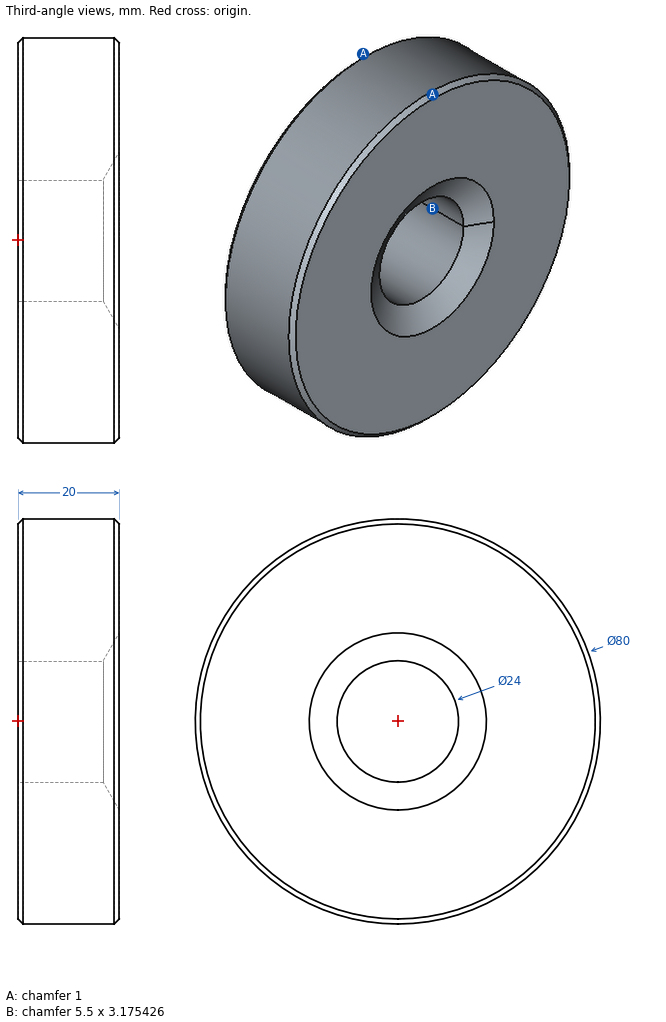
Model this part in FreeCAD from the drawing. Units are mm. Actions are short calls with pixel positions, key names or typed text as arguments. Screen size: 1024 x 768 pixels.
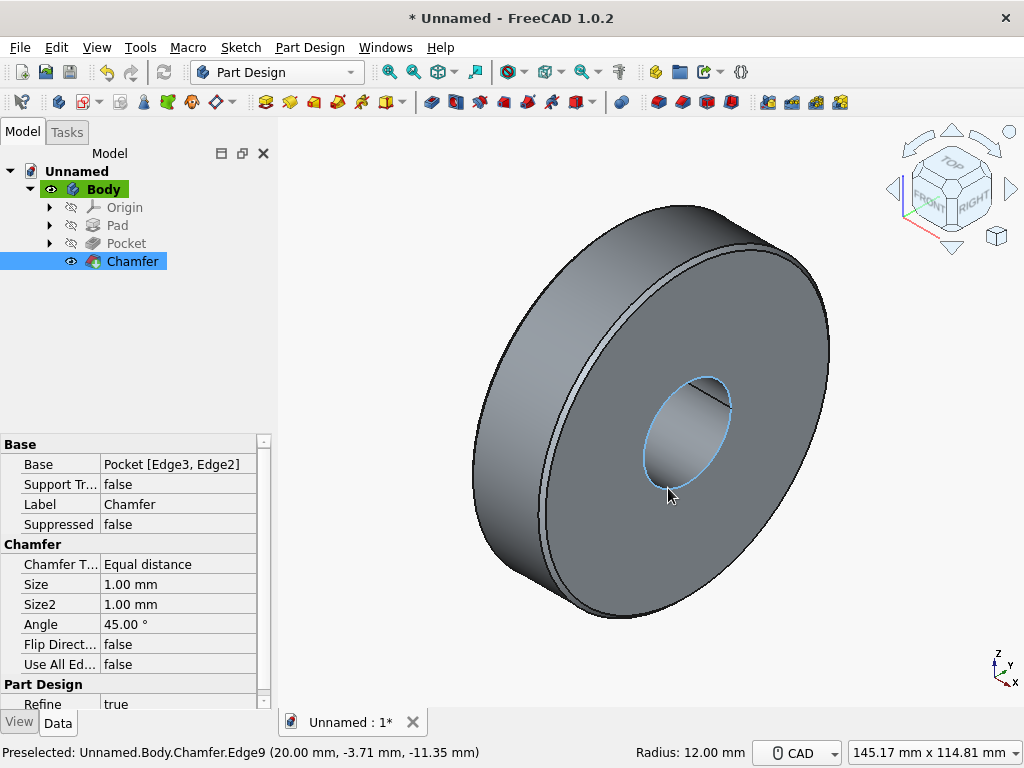
click(684, 102)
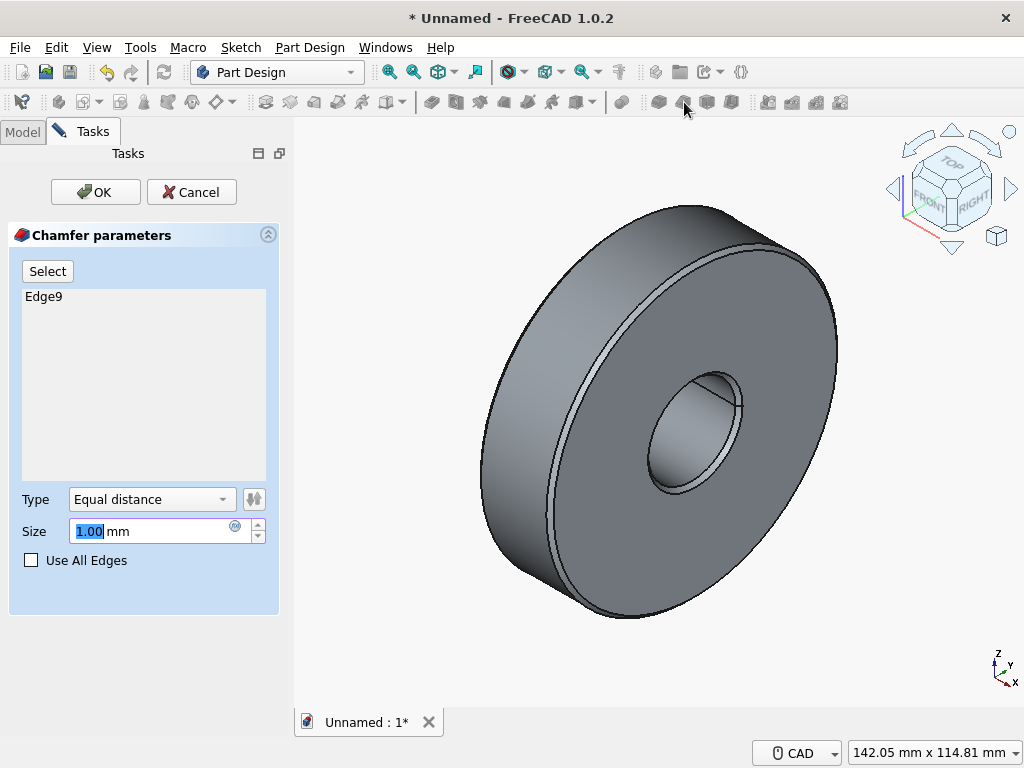
text(5.5)
key(Tab)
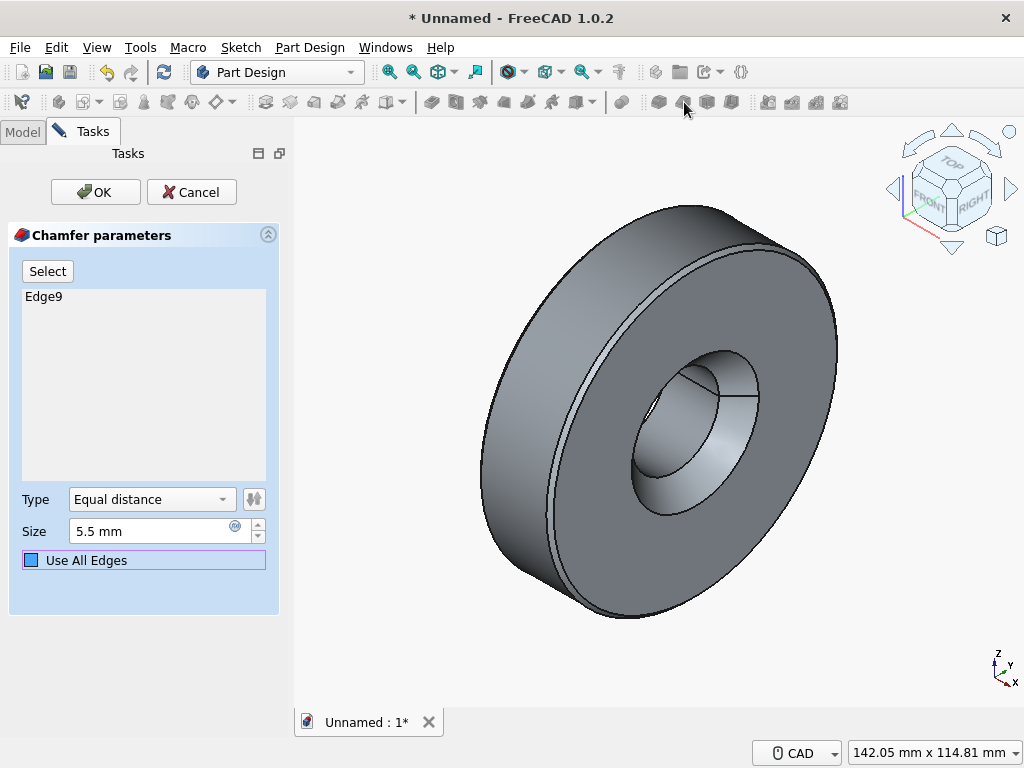
click(153, 500)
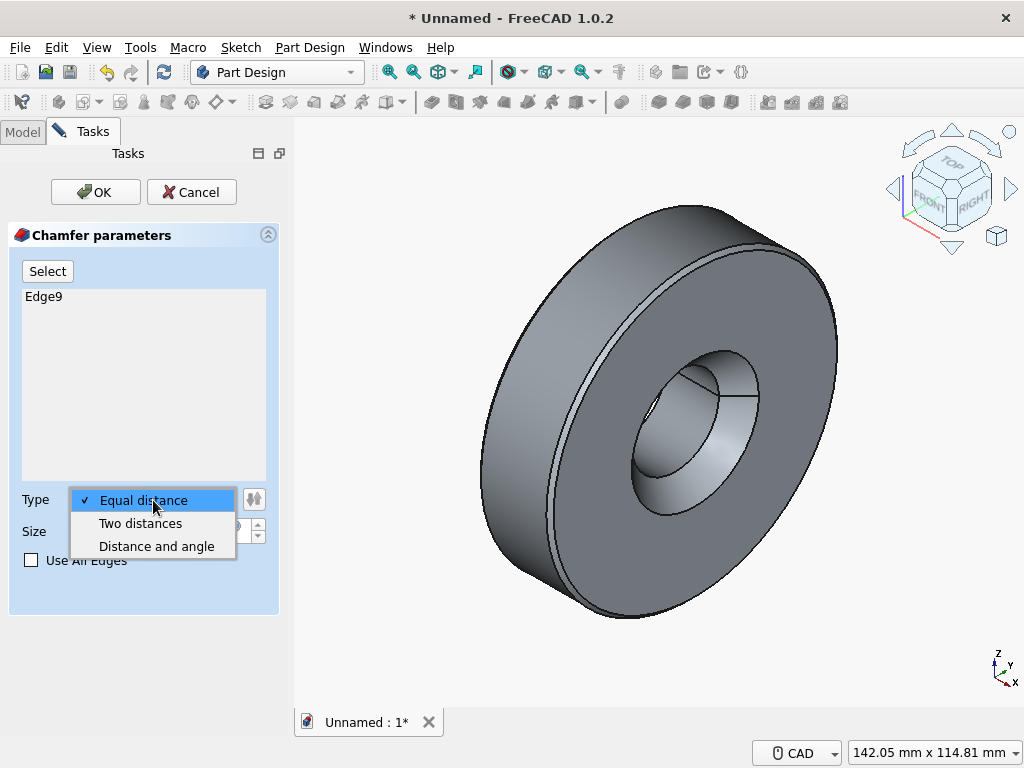
click(152, 524)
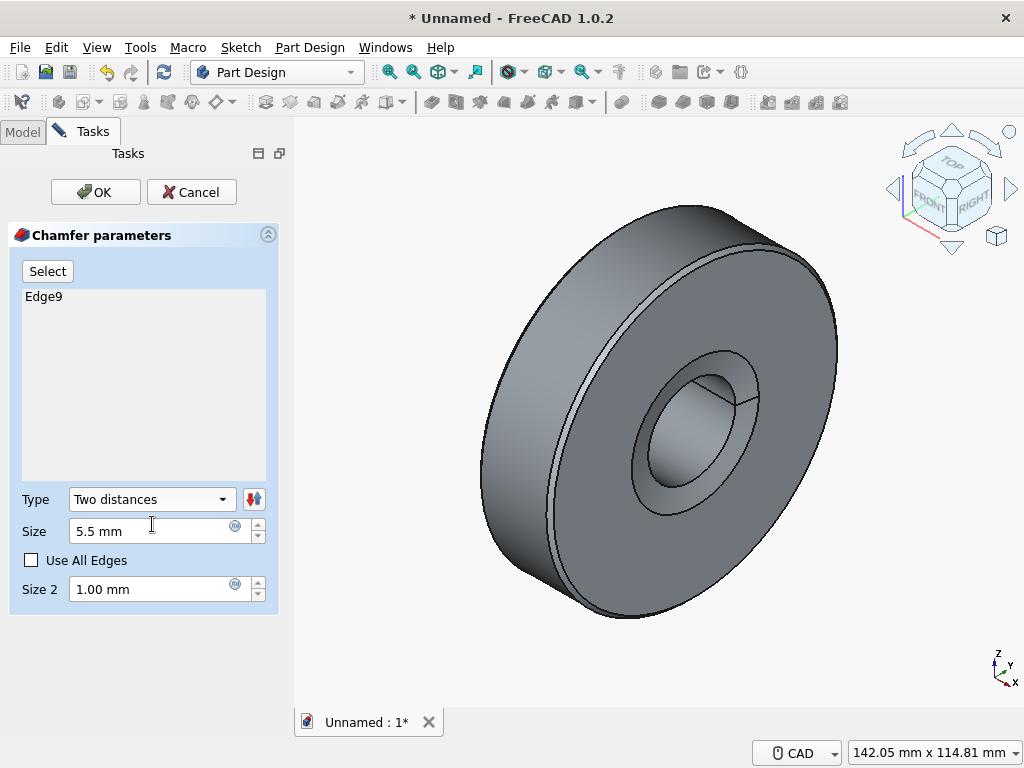
triple_click(160, 589)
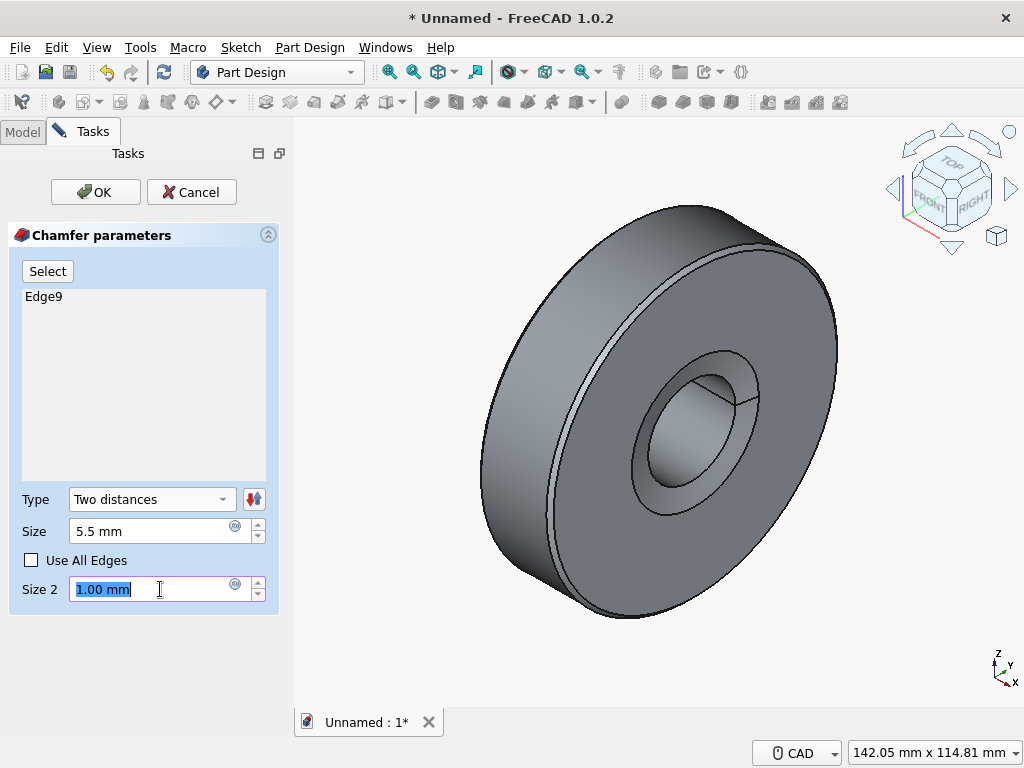
text(3.175426)
key(Tab)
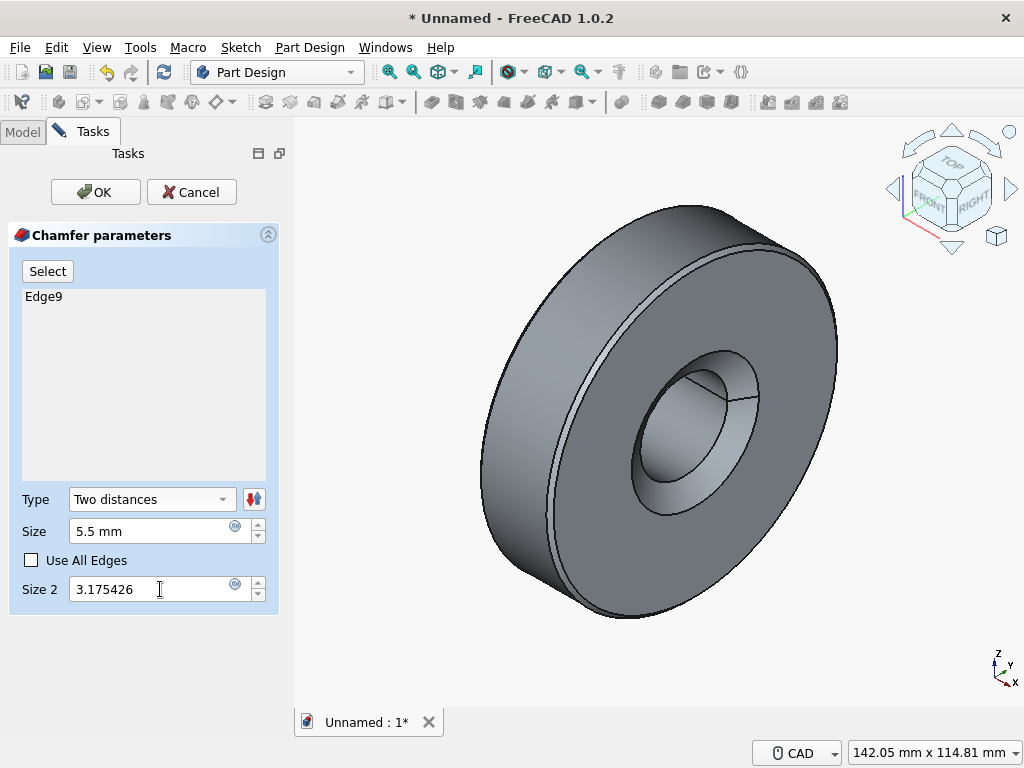
click(96, 192)